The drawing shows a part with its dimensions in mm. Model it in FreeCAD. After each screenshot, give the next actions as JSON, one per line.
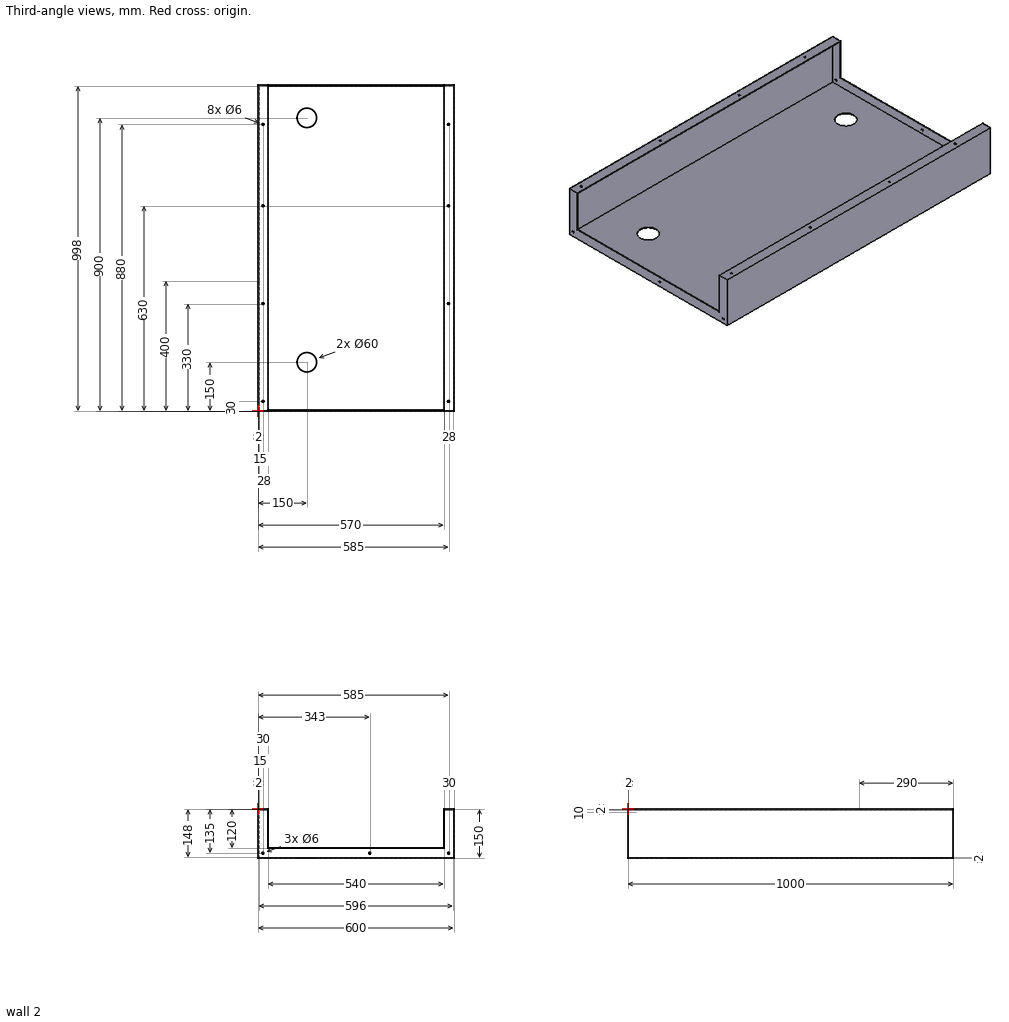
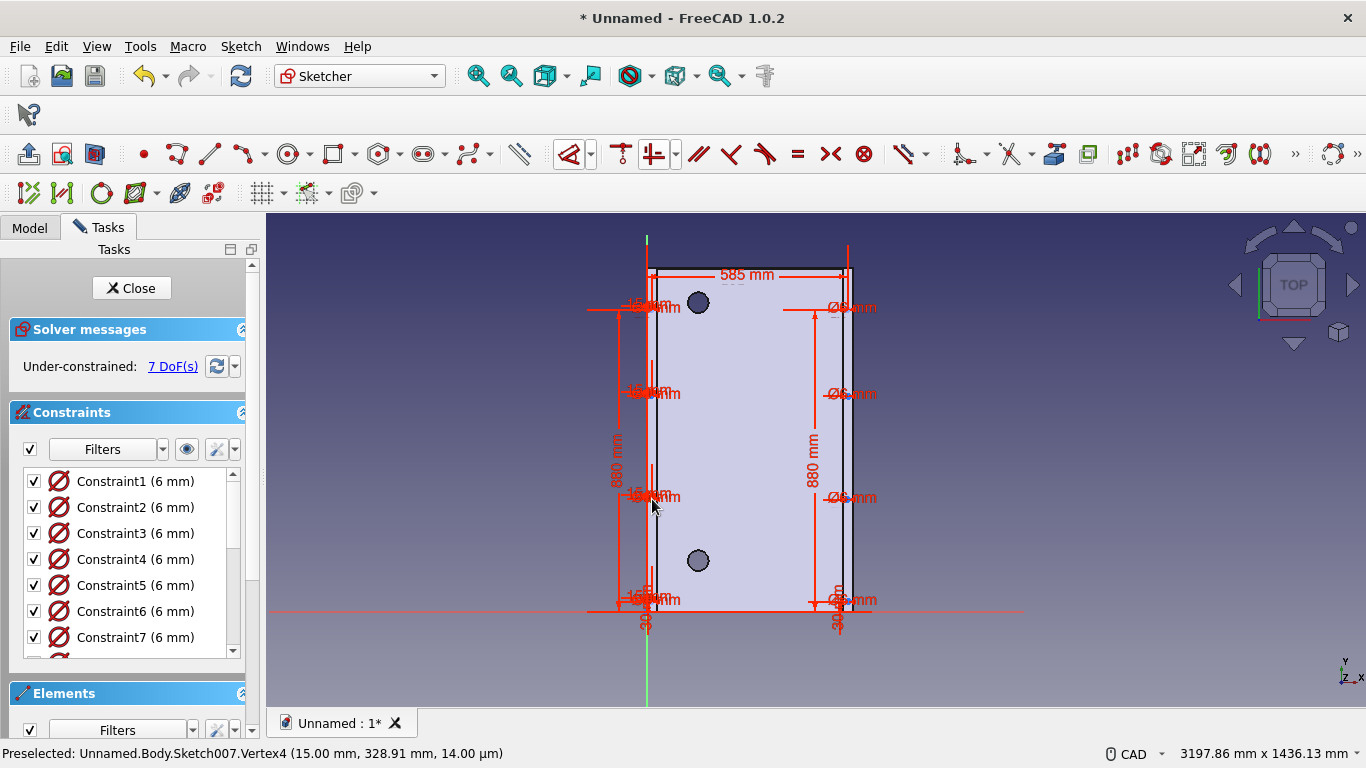
{"action": "left_click", "coordinate": [590, 154]}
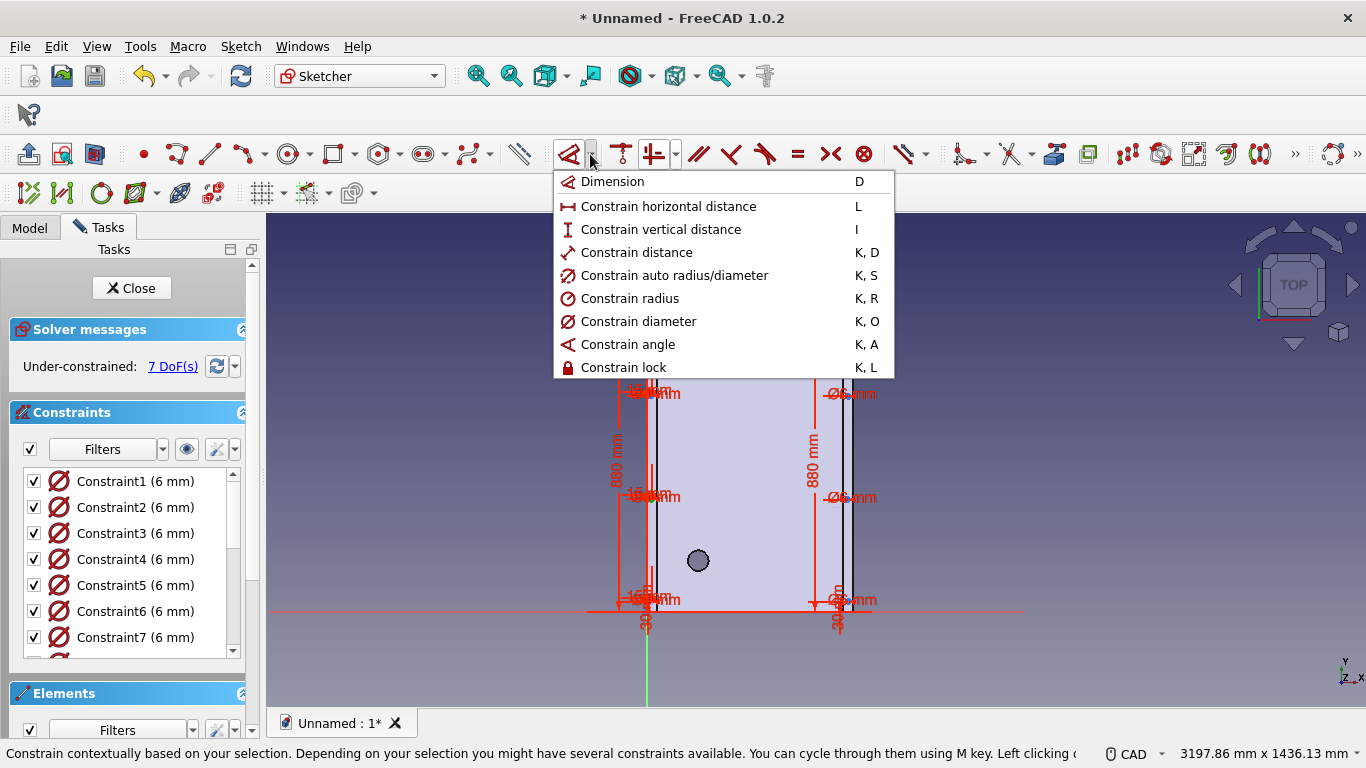
{"action": "left_click", "coordinate": [724, 230]}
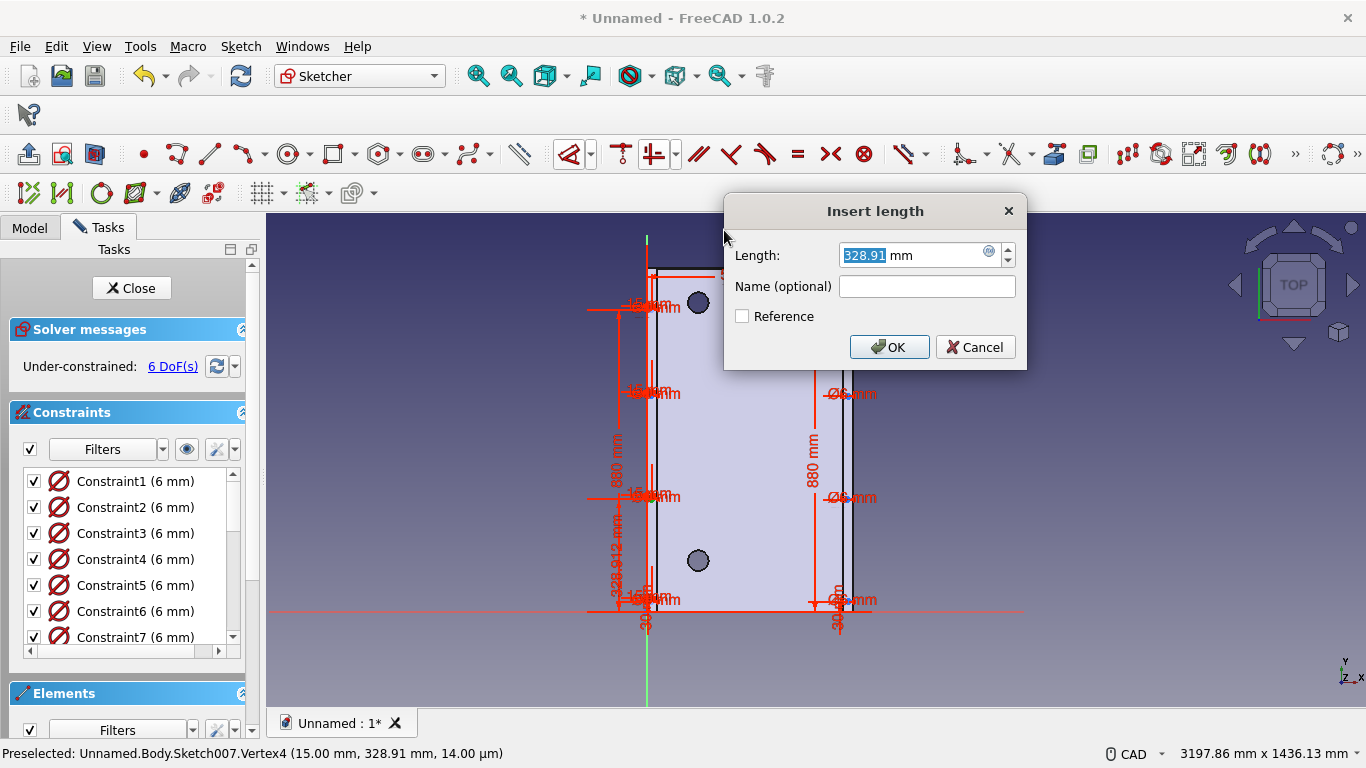
{"action": "type", "text": "330"}
{"action": "key", "text": "Return"}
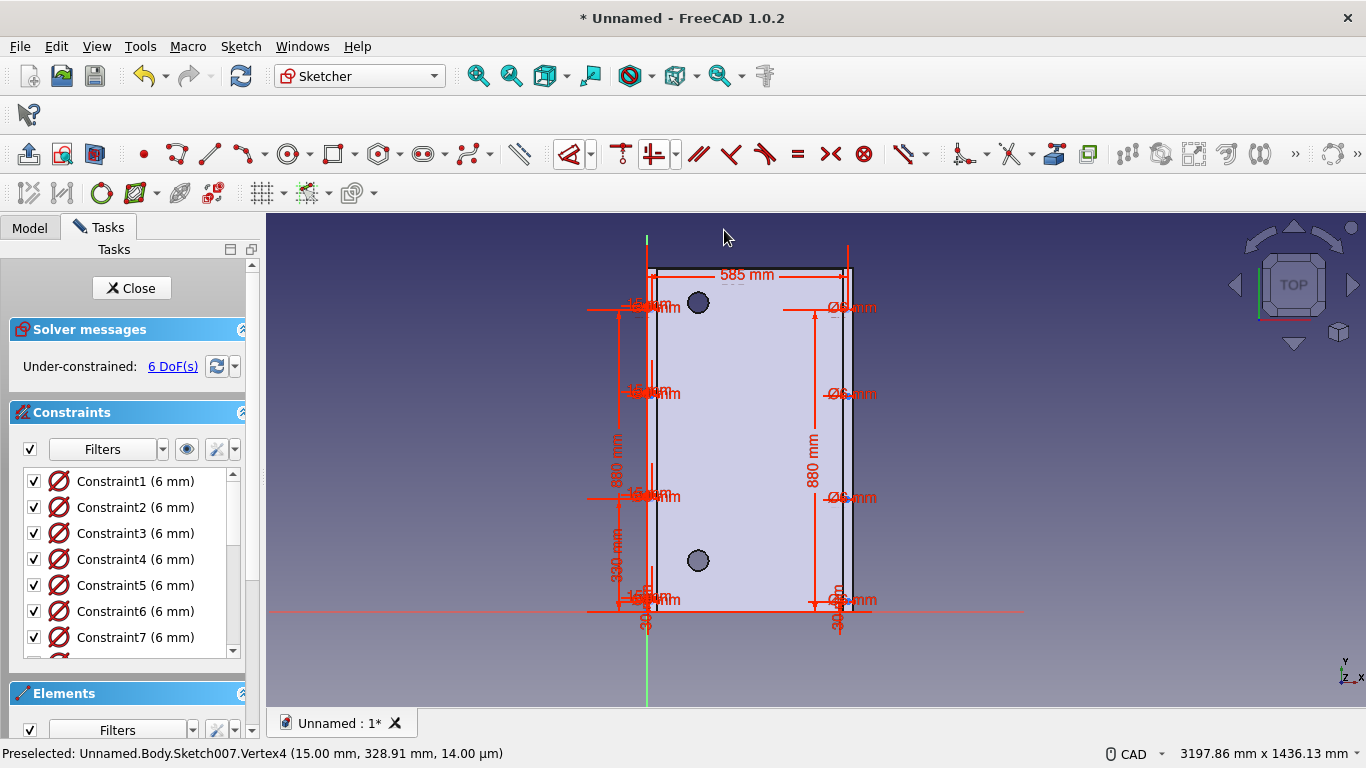
{"action": "left_click", "coordinate": [848, 396]}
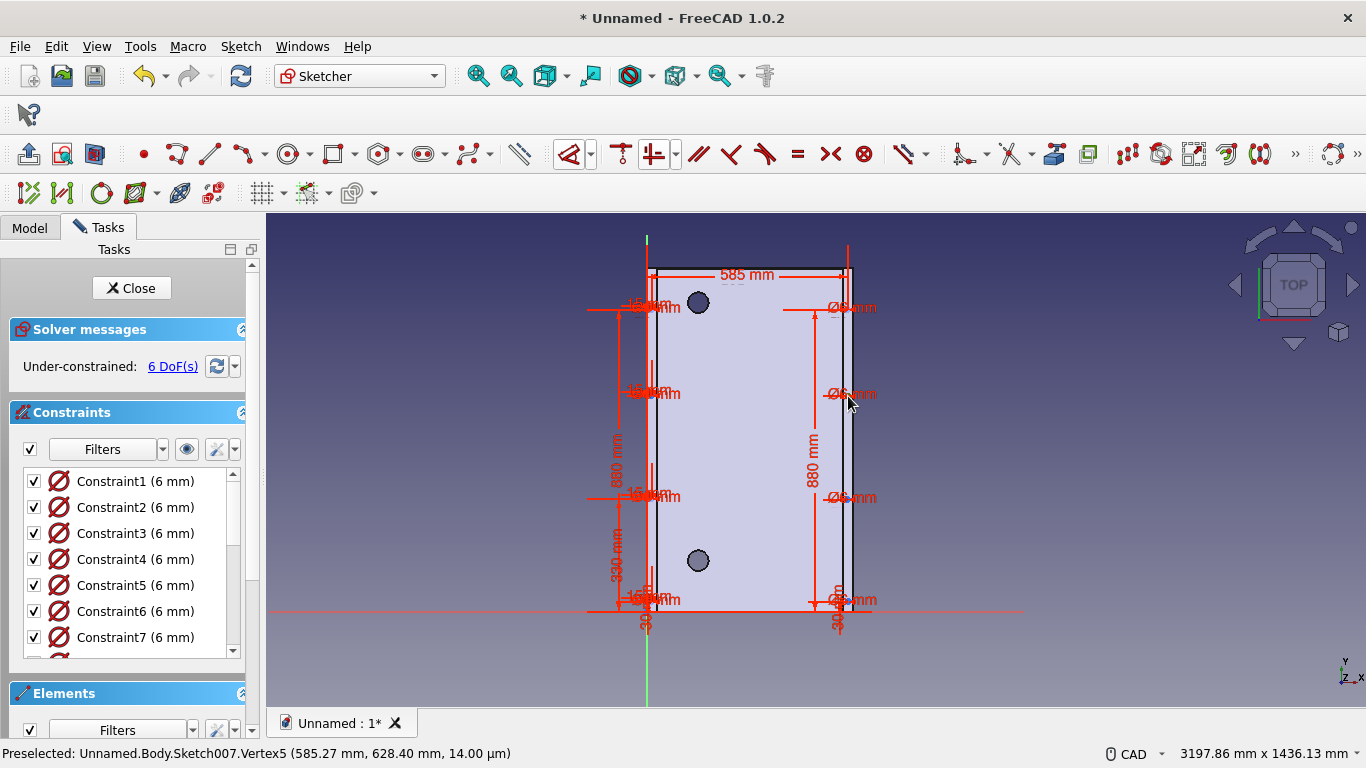
{"action": "left_click", "coordinate": [590, 154]}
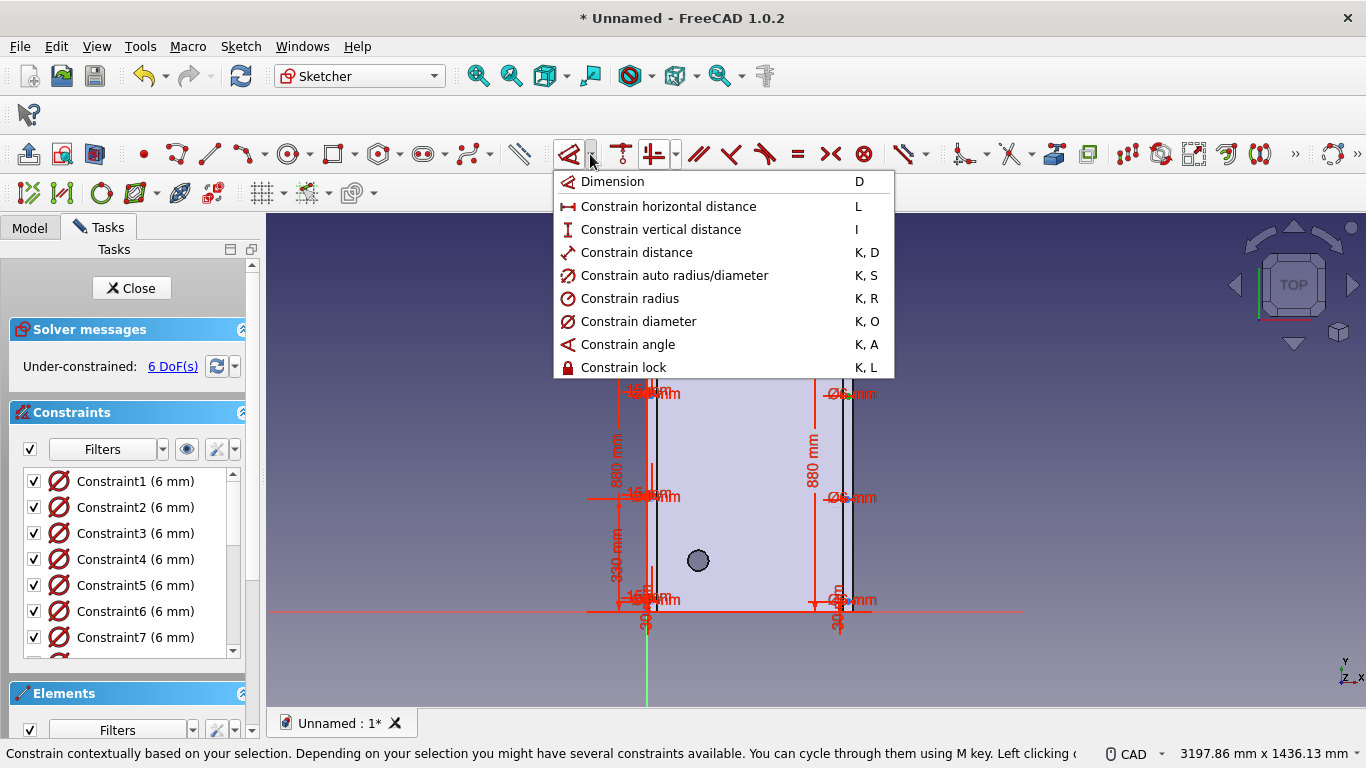
{"action": "left_click", "coordinate": [724, 206]}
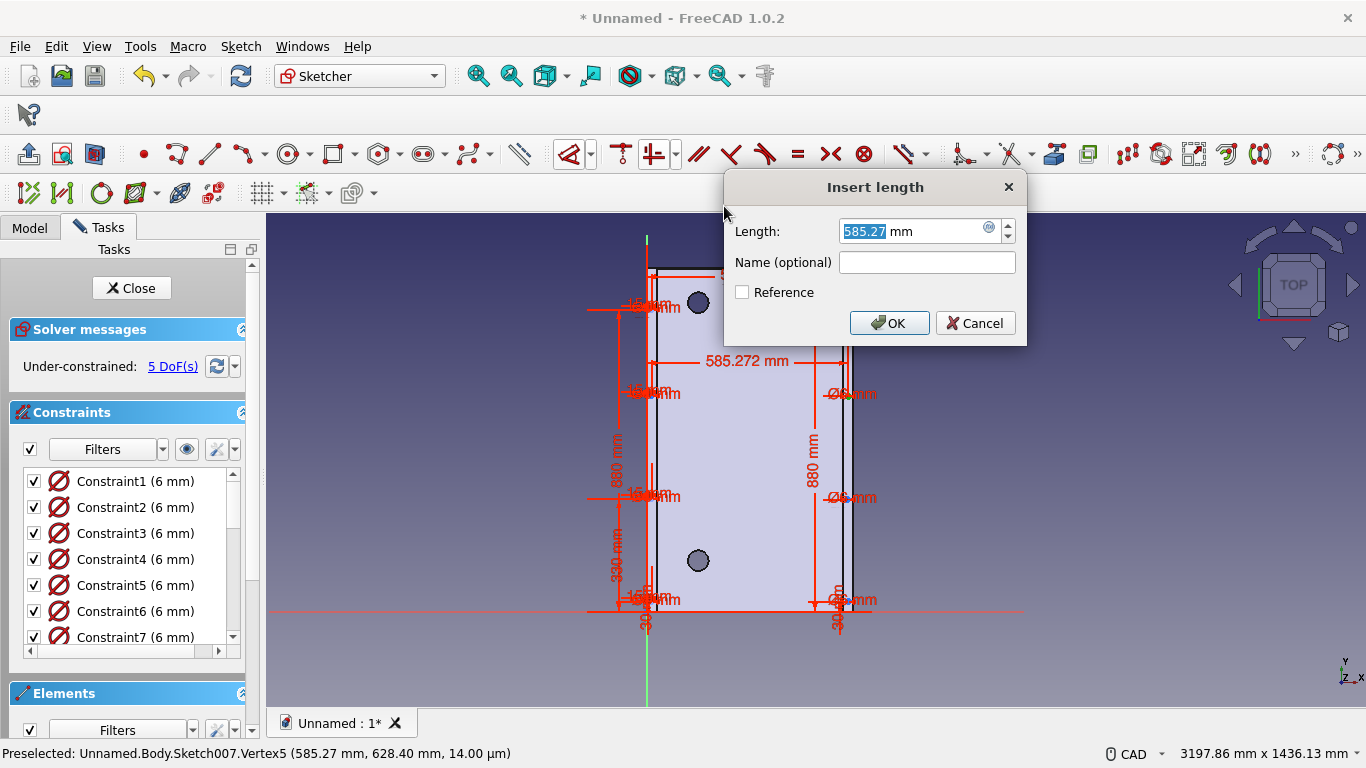
{"action": "type", "text": "585"}
{"action": "key", "text": "Return"}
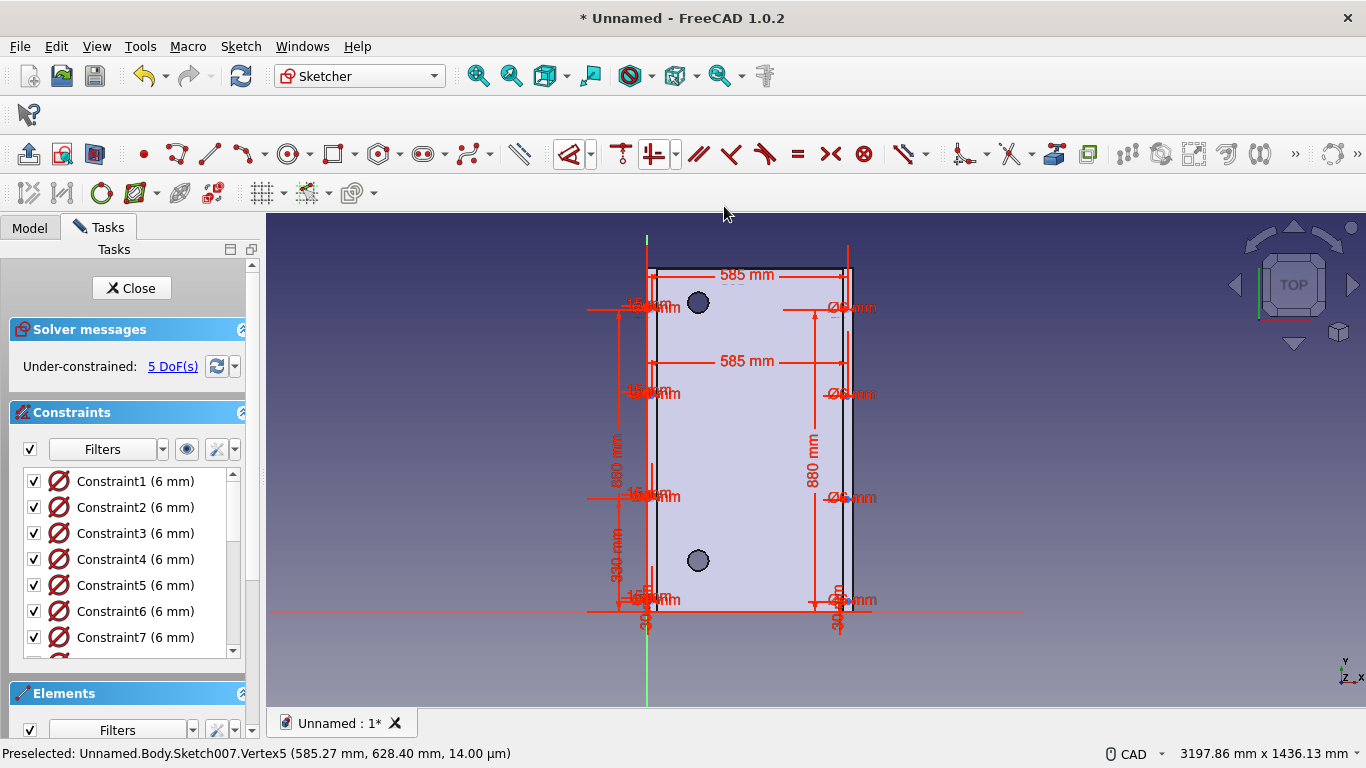
{"action": "left_click", "coordinate": [848, 396]}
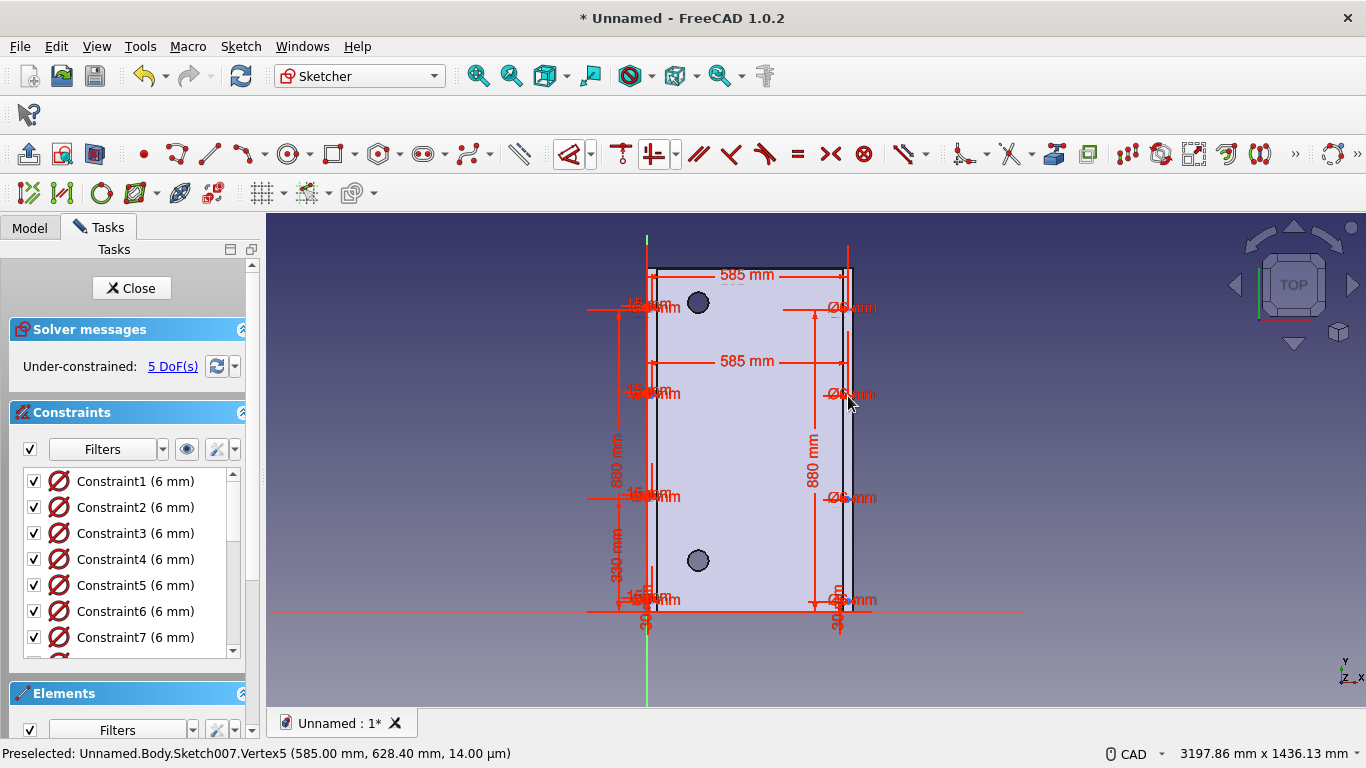
{"action": "key", "text": "i"}